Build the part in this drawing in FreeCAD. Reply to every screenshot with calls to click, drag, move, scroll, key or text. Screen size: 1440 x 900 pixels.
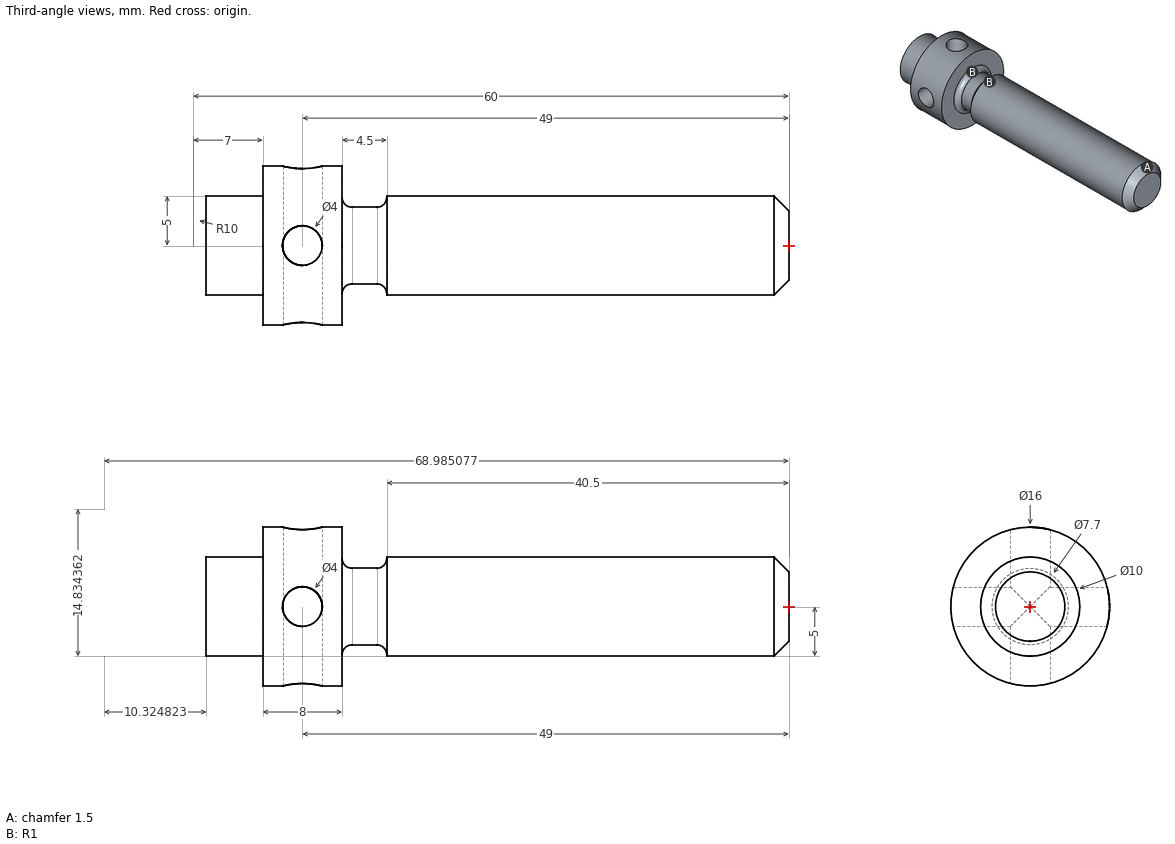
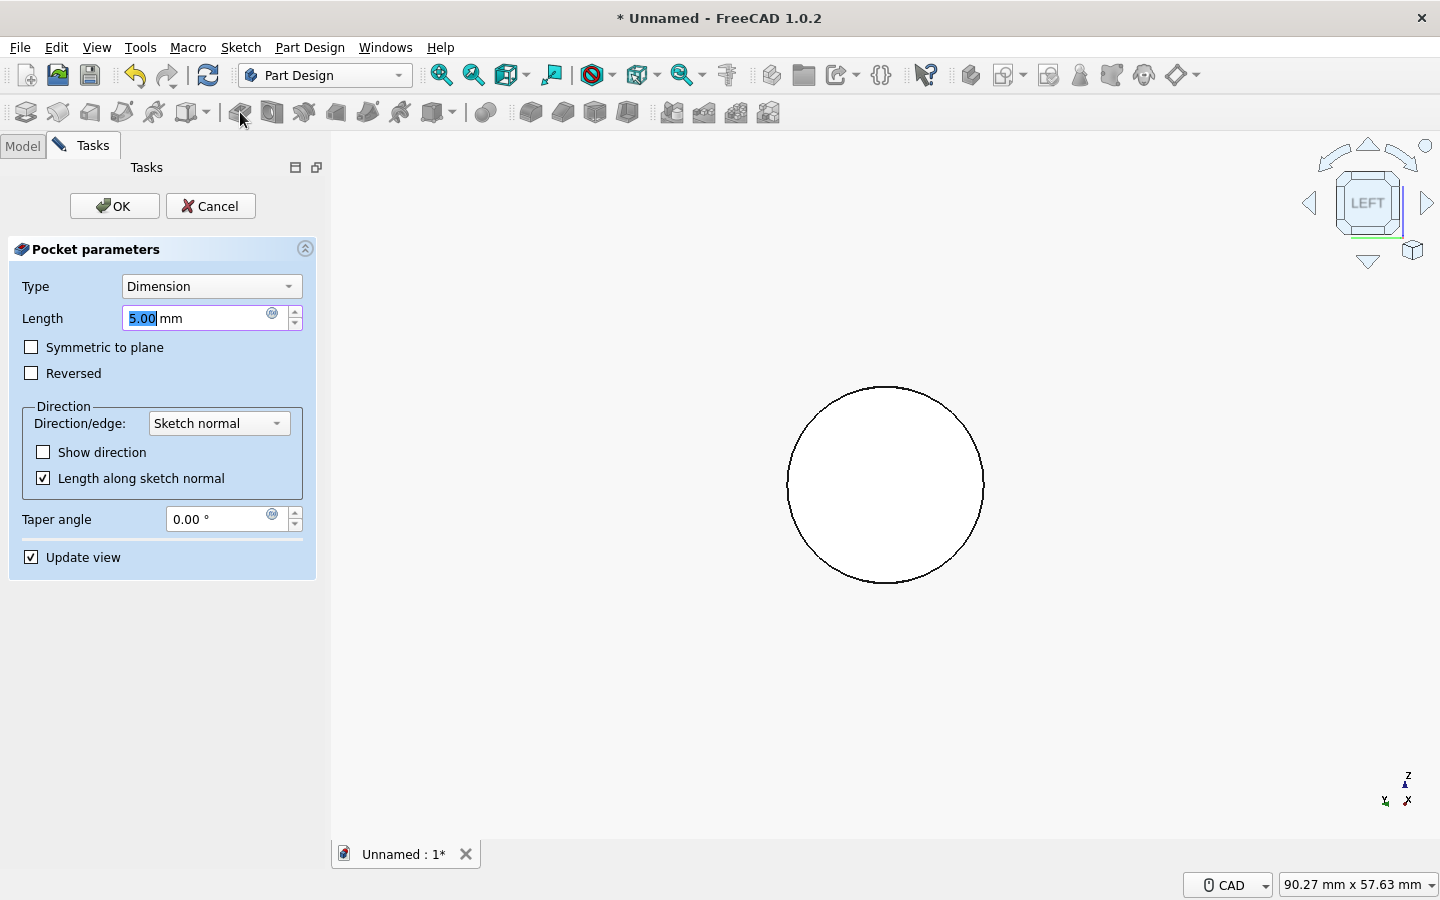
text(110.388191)
key(Tab)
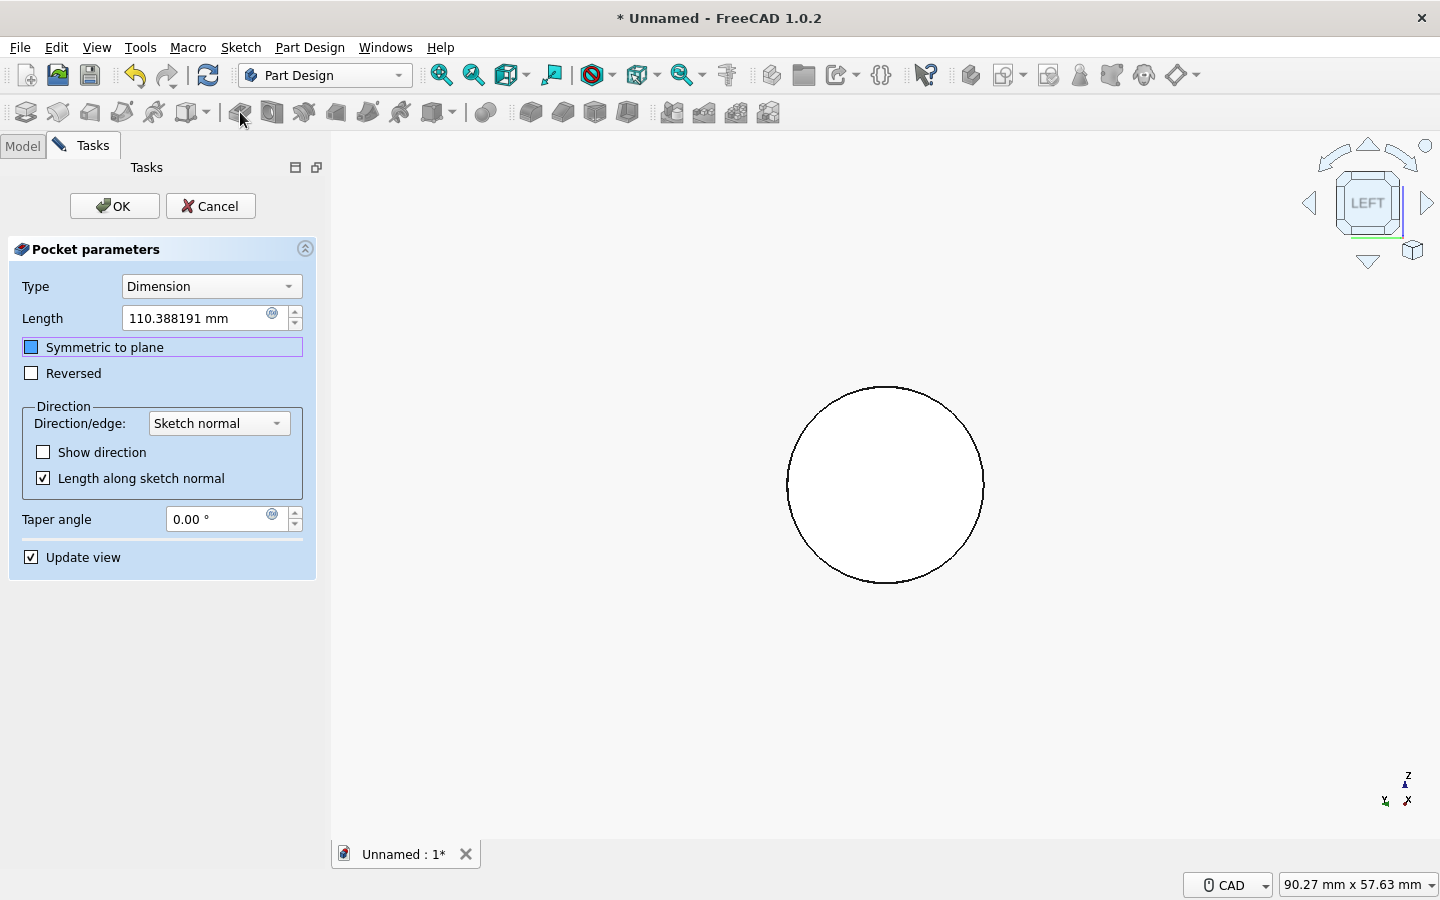
click(30, 347)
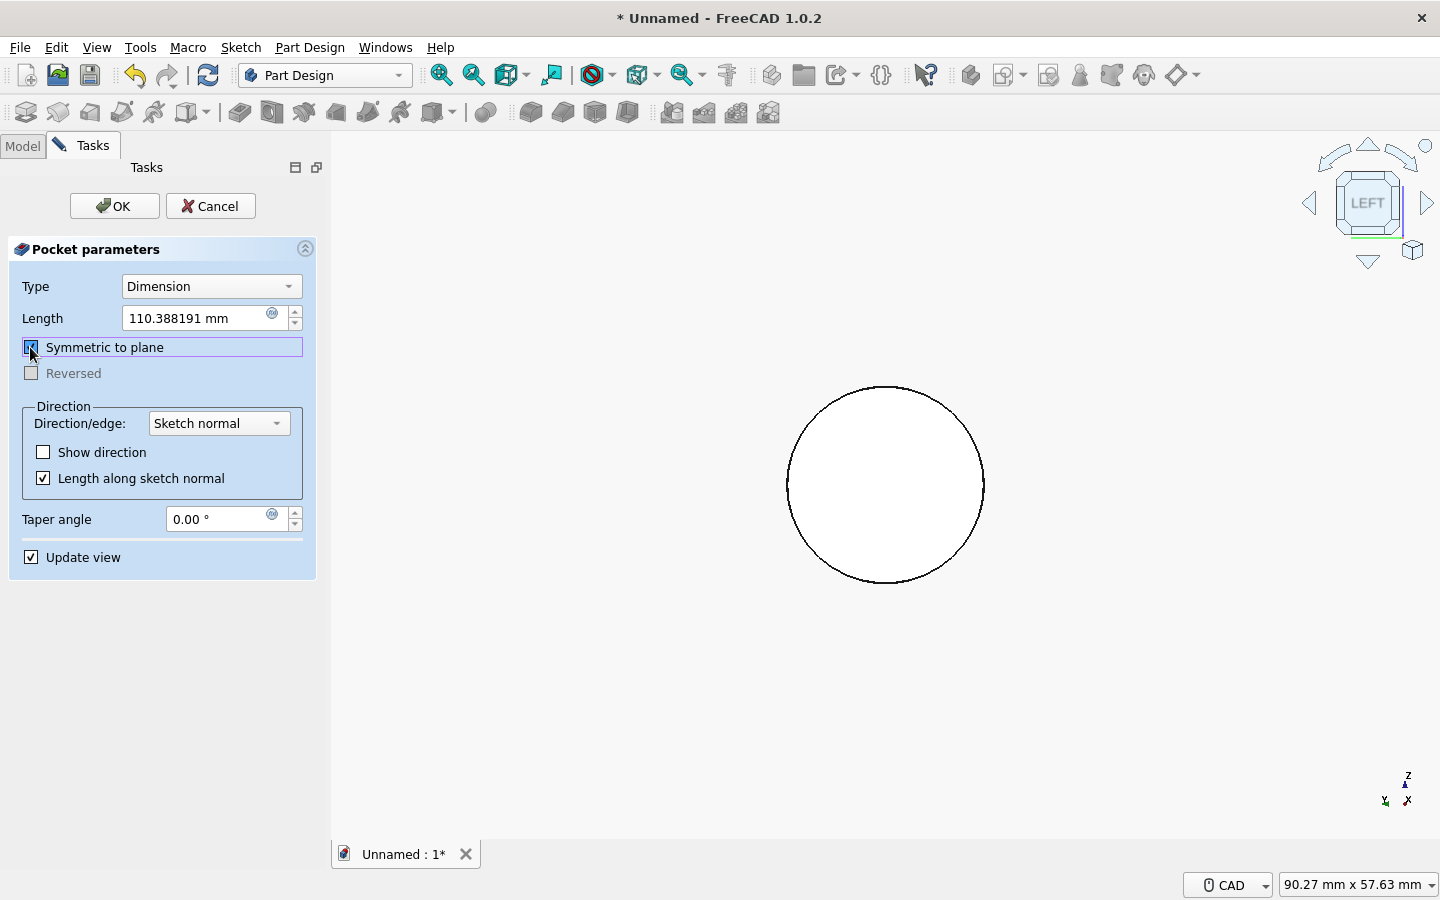
click(115, 206)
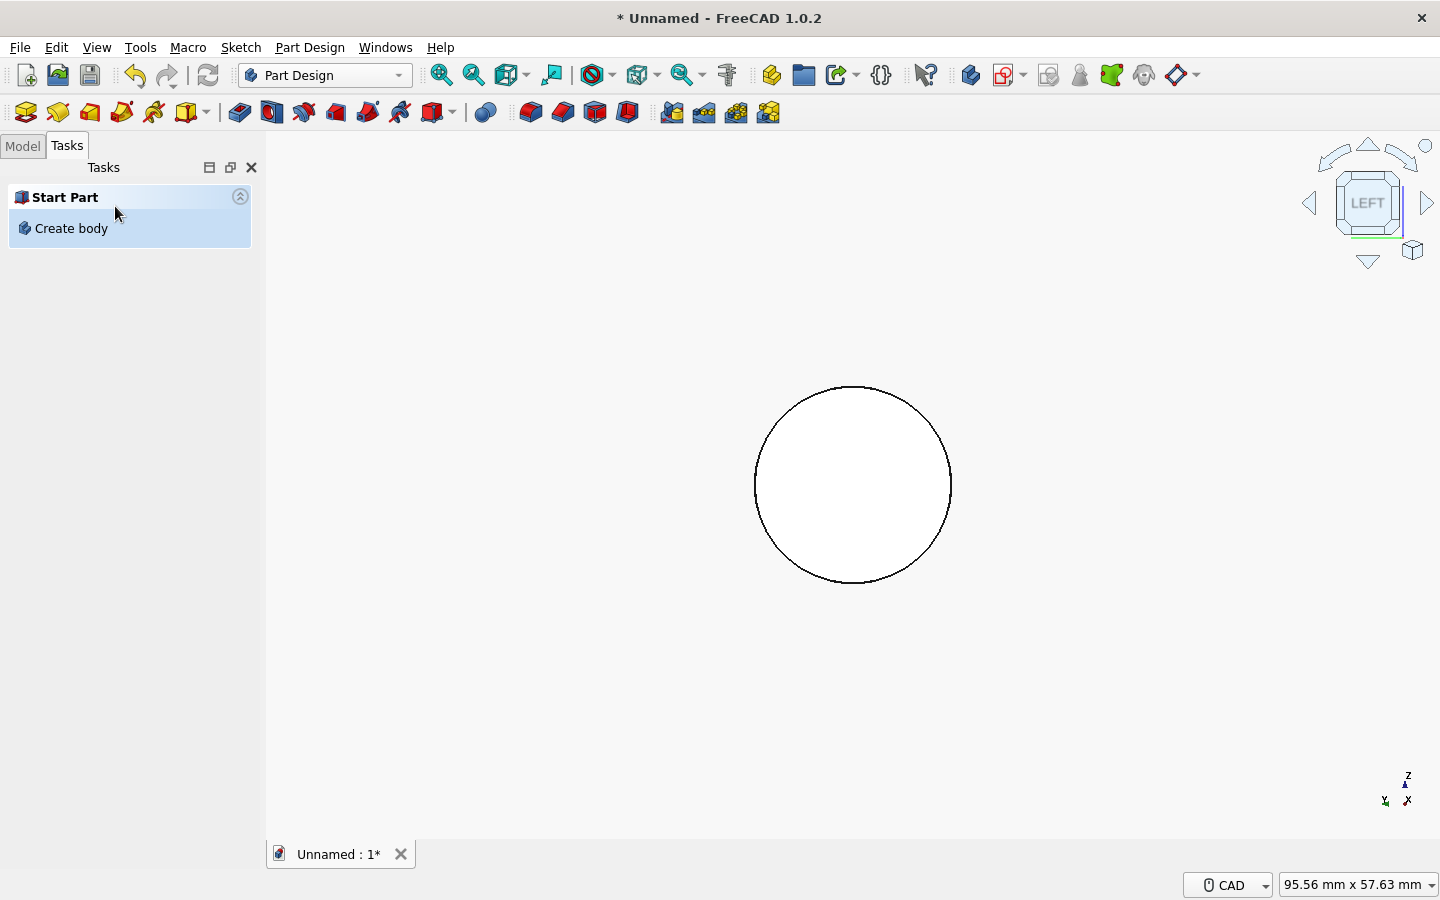
click(442, 76)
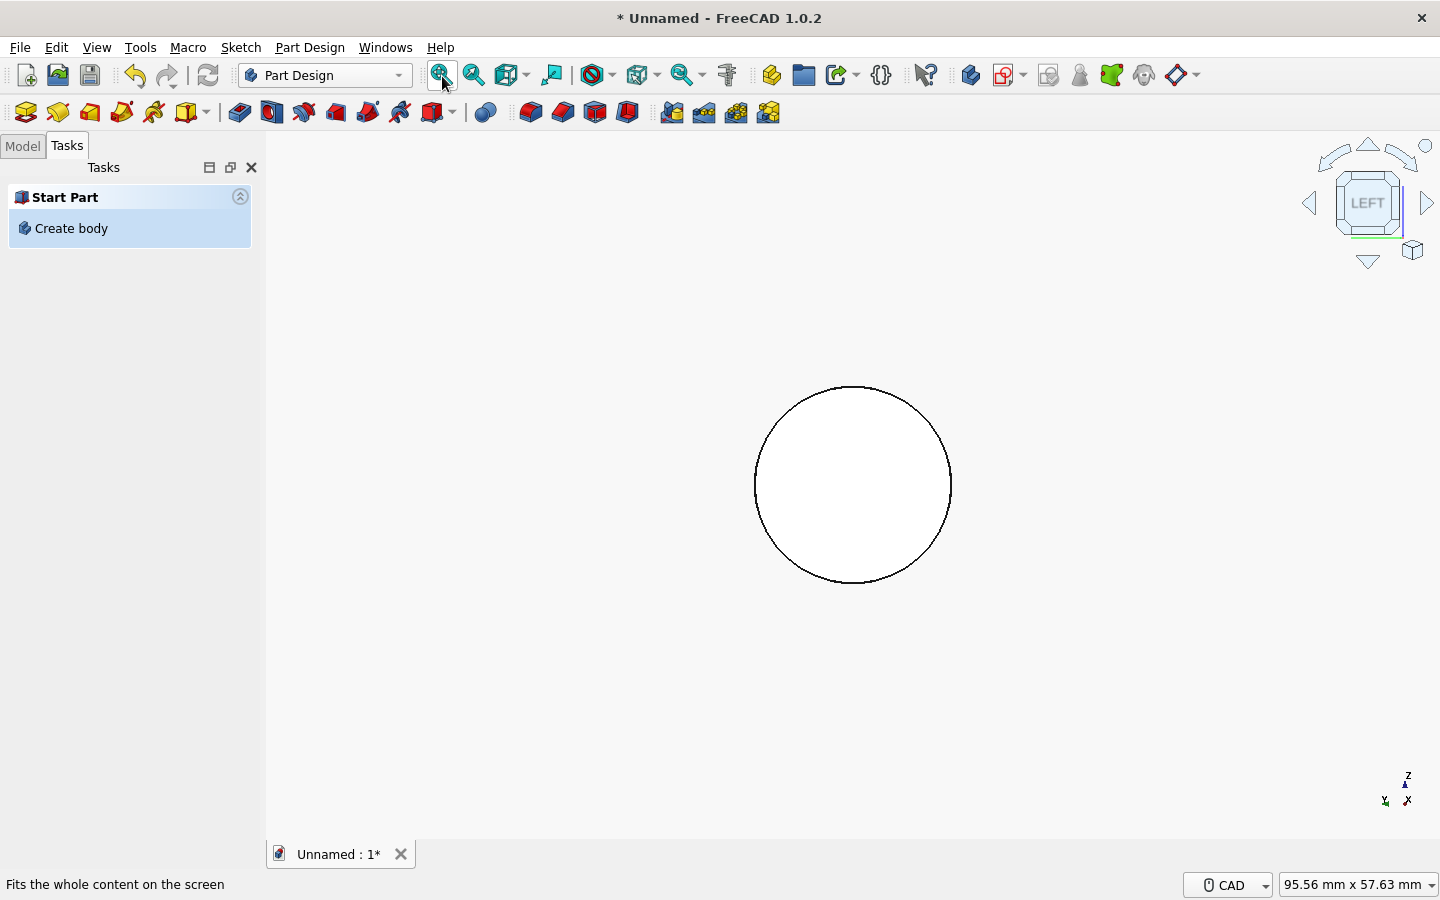
click(1004, 76)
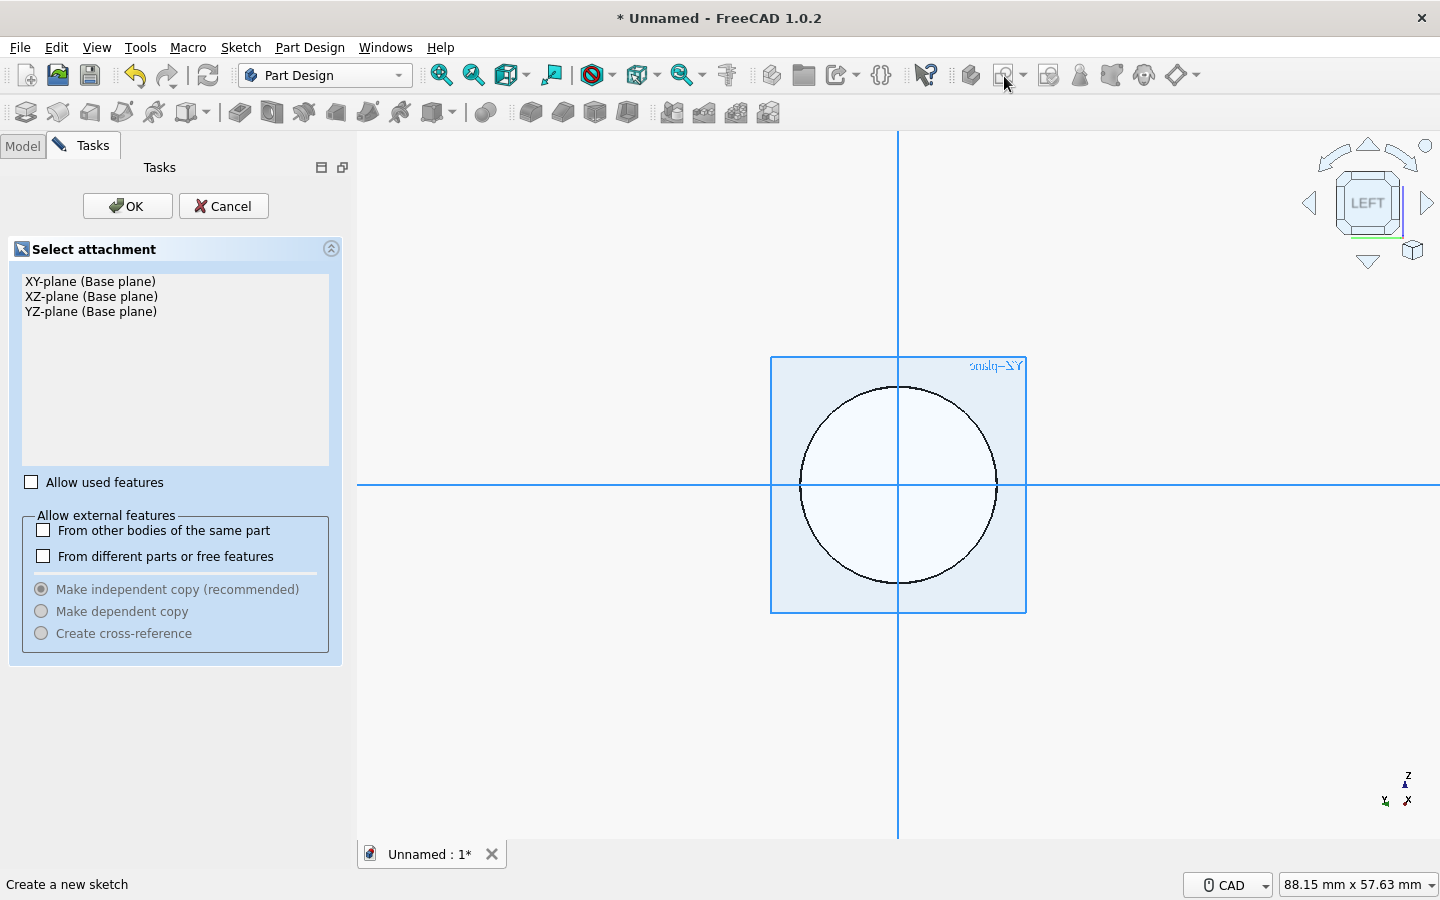
click(82, 282)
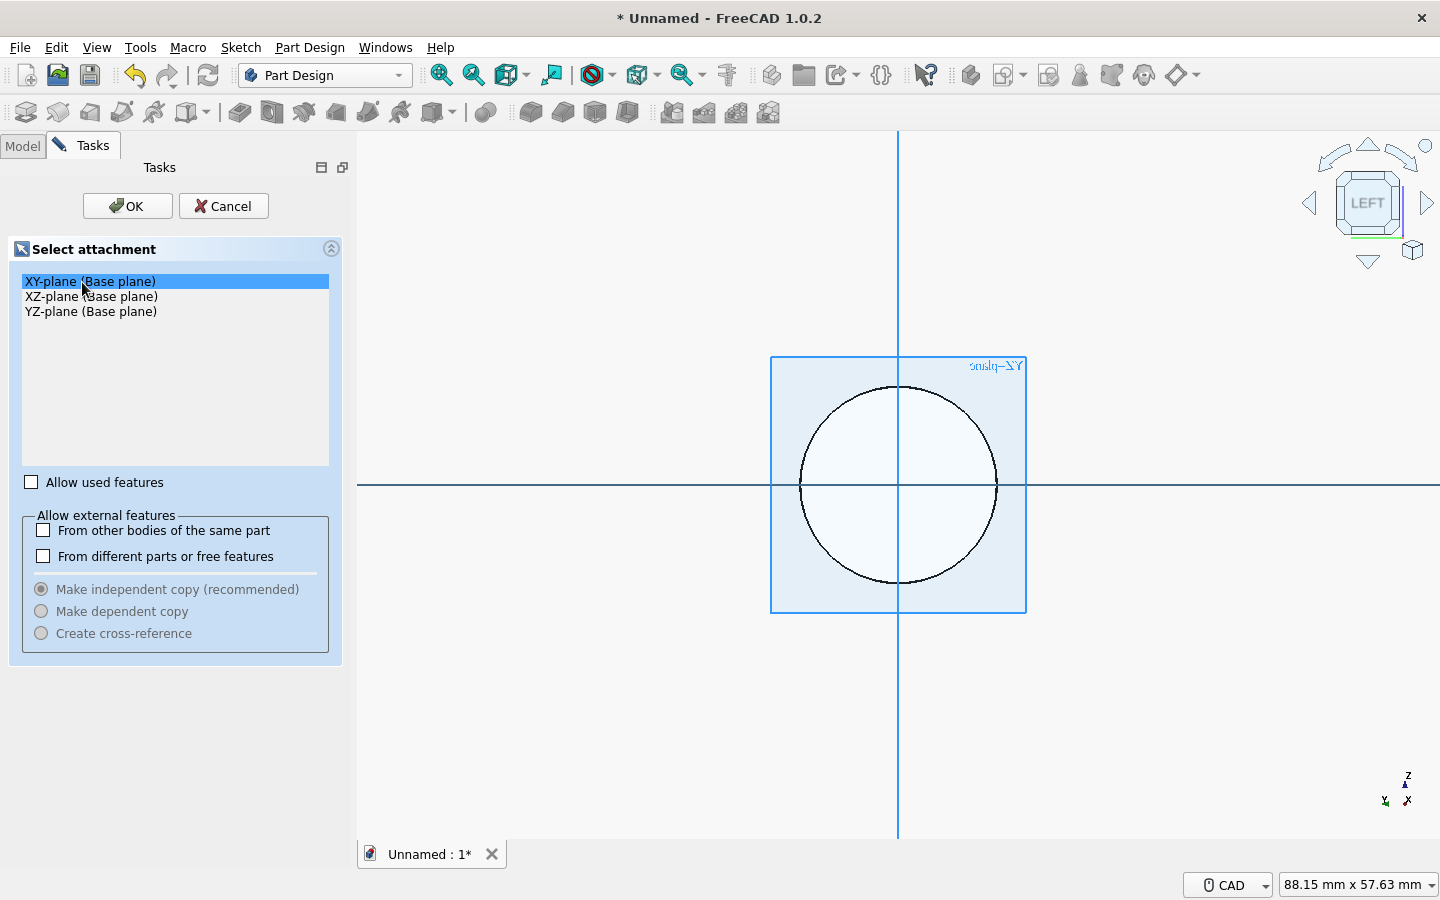
click(128, 206)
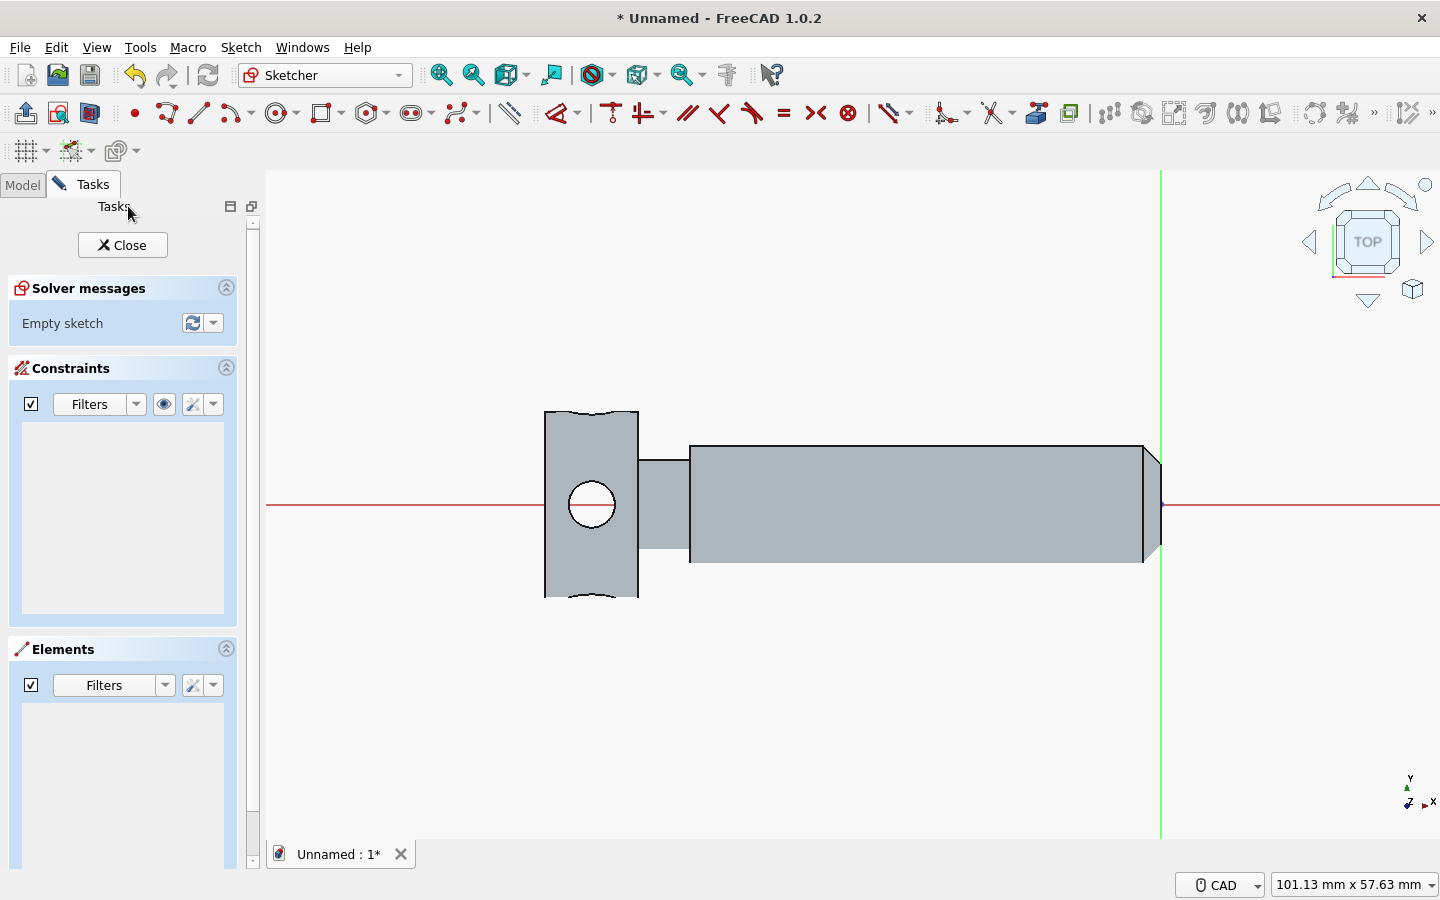
key(q)
key(s)